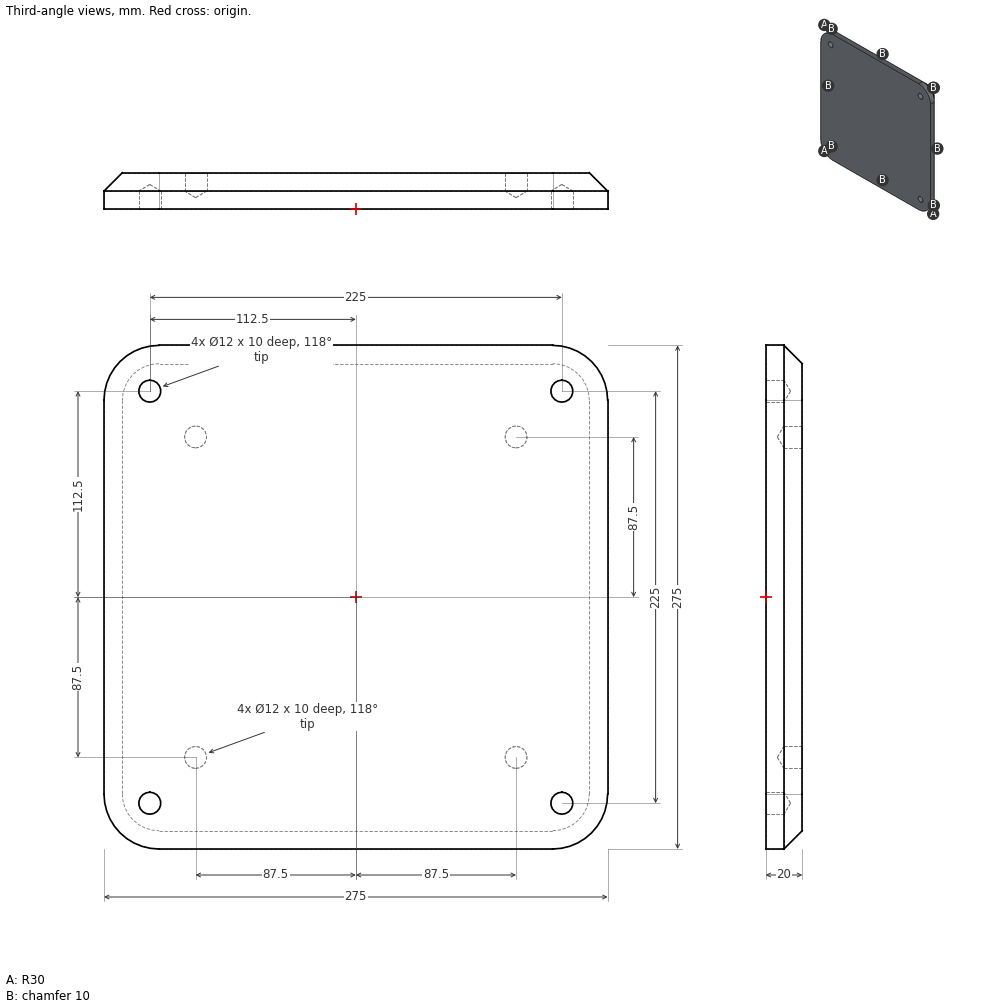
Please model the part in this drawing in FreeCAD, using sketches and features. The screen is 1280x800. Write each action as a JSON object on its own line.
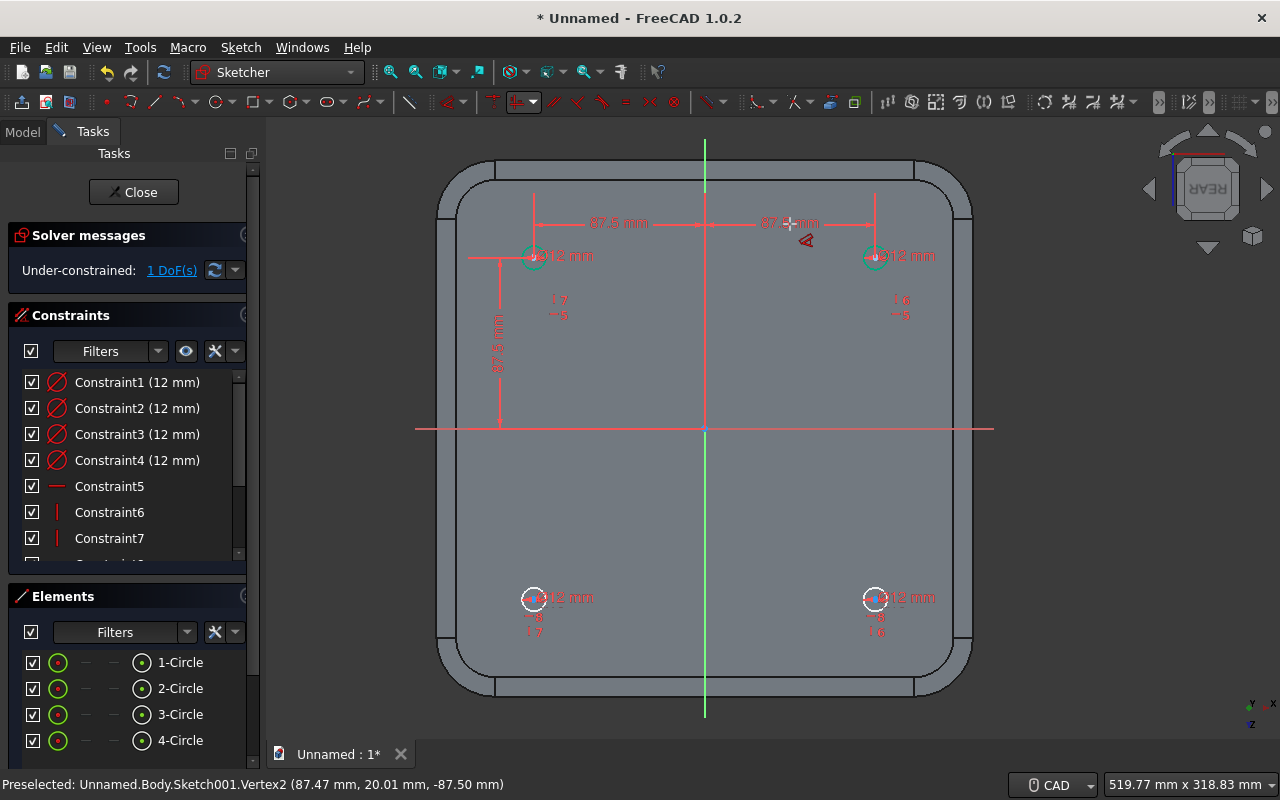
{"action": "left_click", "coordinate": [875, 600]}
{"action": "left_click", "coordinate": [909, 514]}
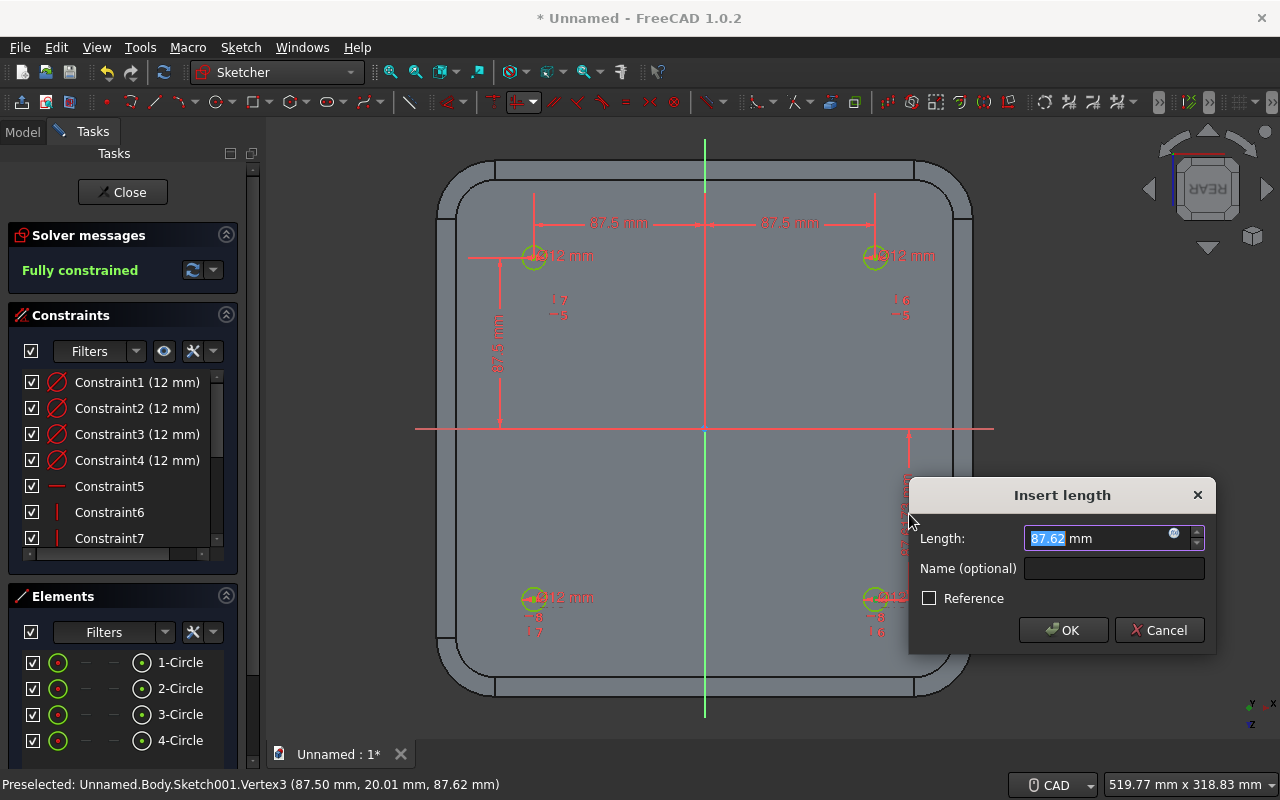
{"action": "type", "text": "87.5"}
{"action": "key", "text": "Return"}
{"action": "key", "text": "Escape"}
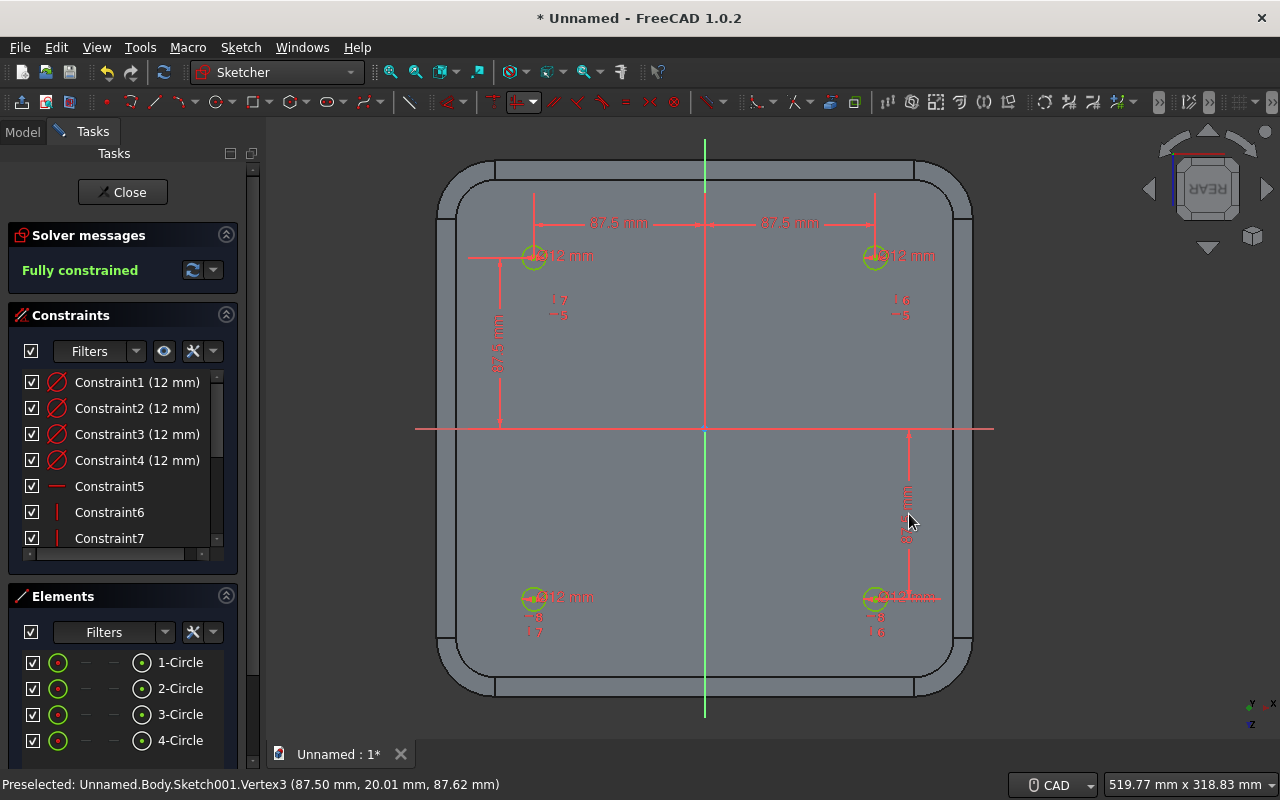
{"action": "left_click", "coordinate": [123, 192]}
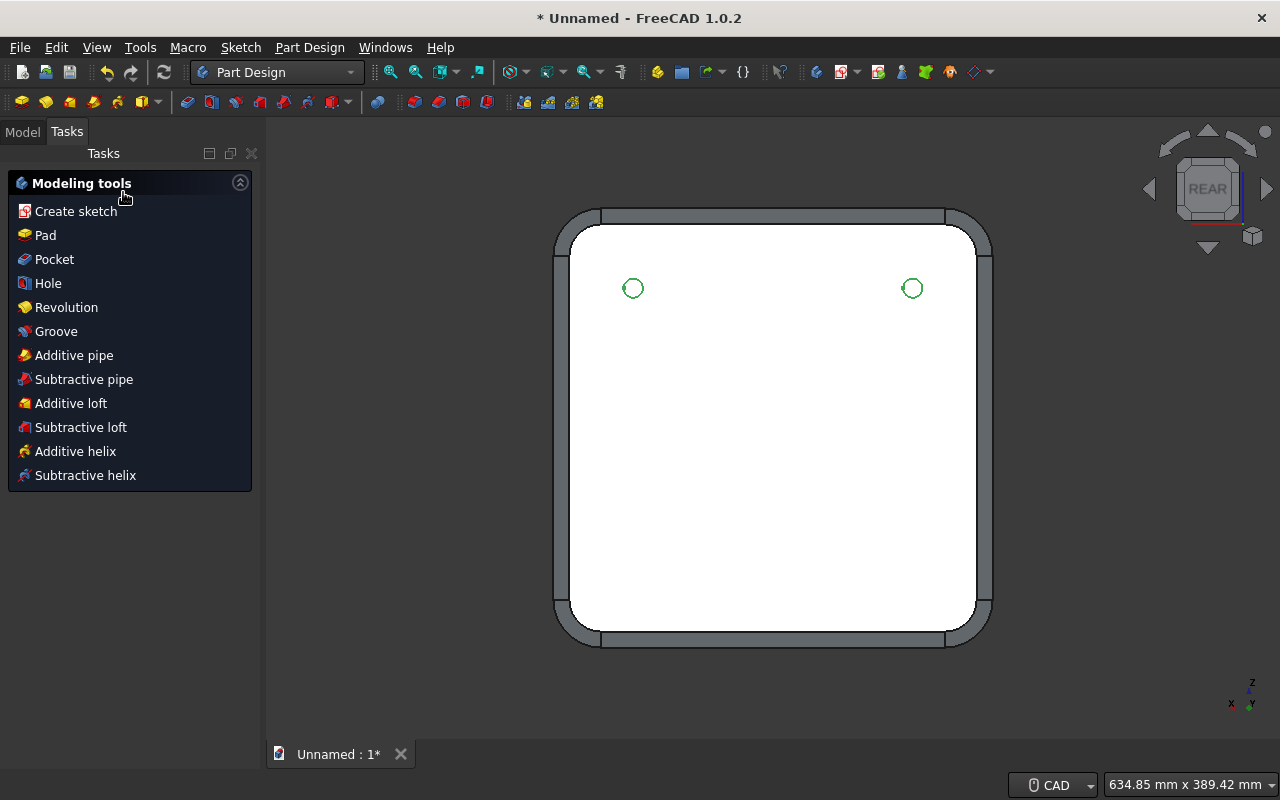
{"action": "left_click", "coordinate": [212, 102]}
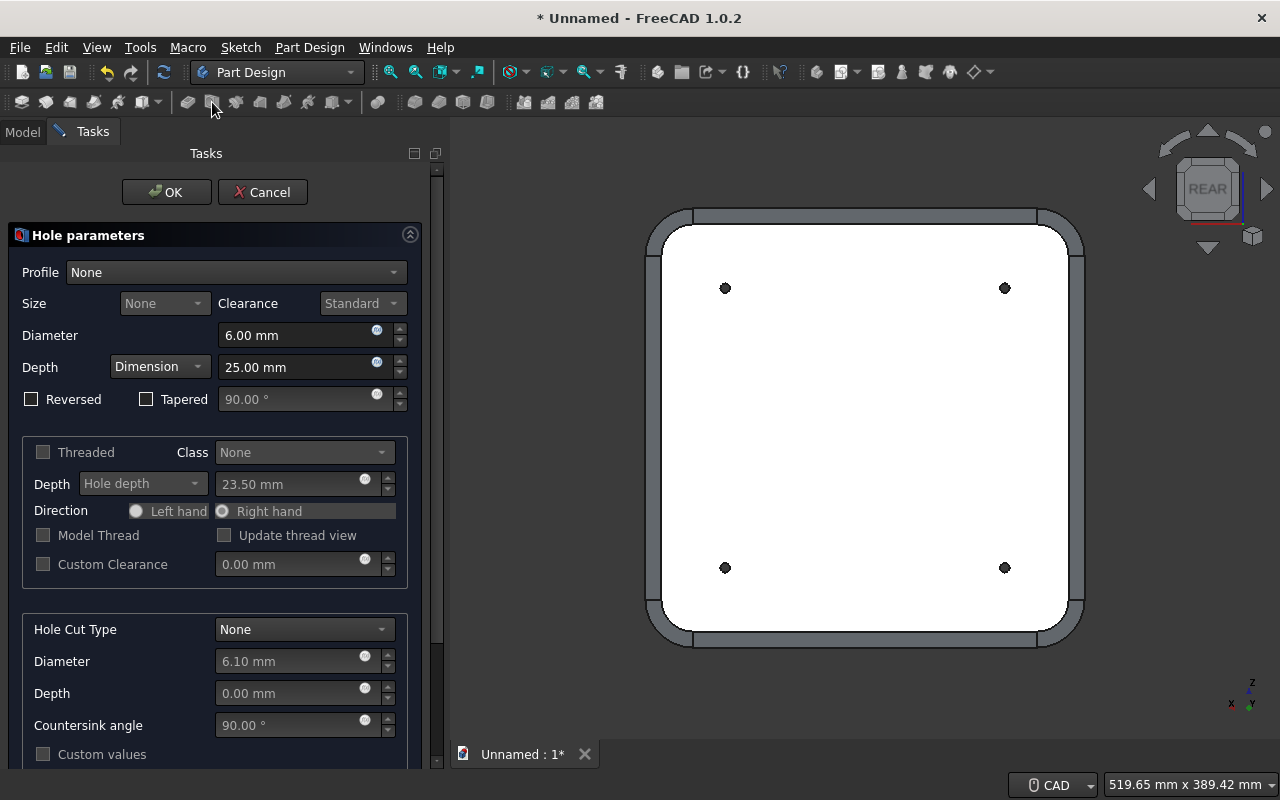
{"action": "triple_click", "coordinate": [305, 335]}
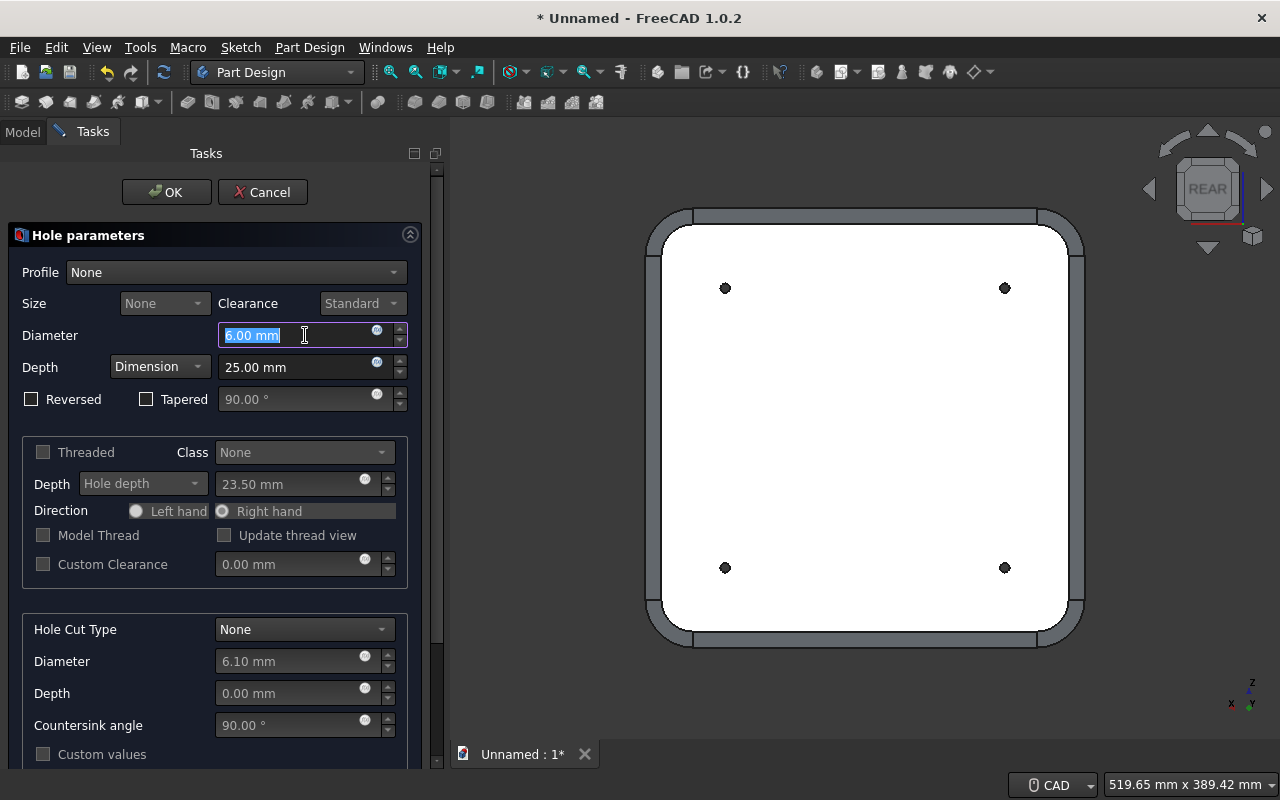
{"action": "type", "text": "12"}
{"action": "key", "text": "Tab"}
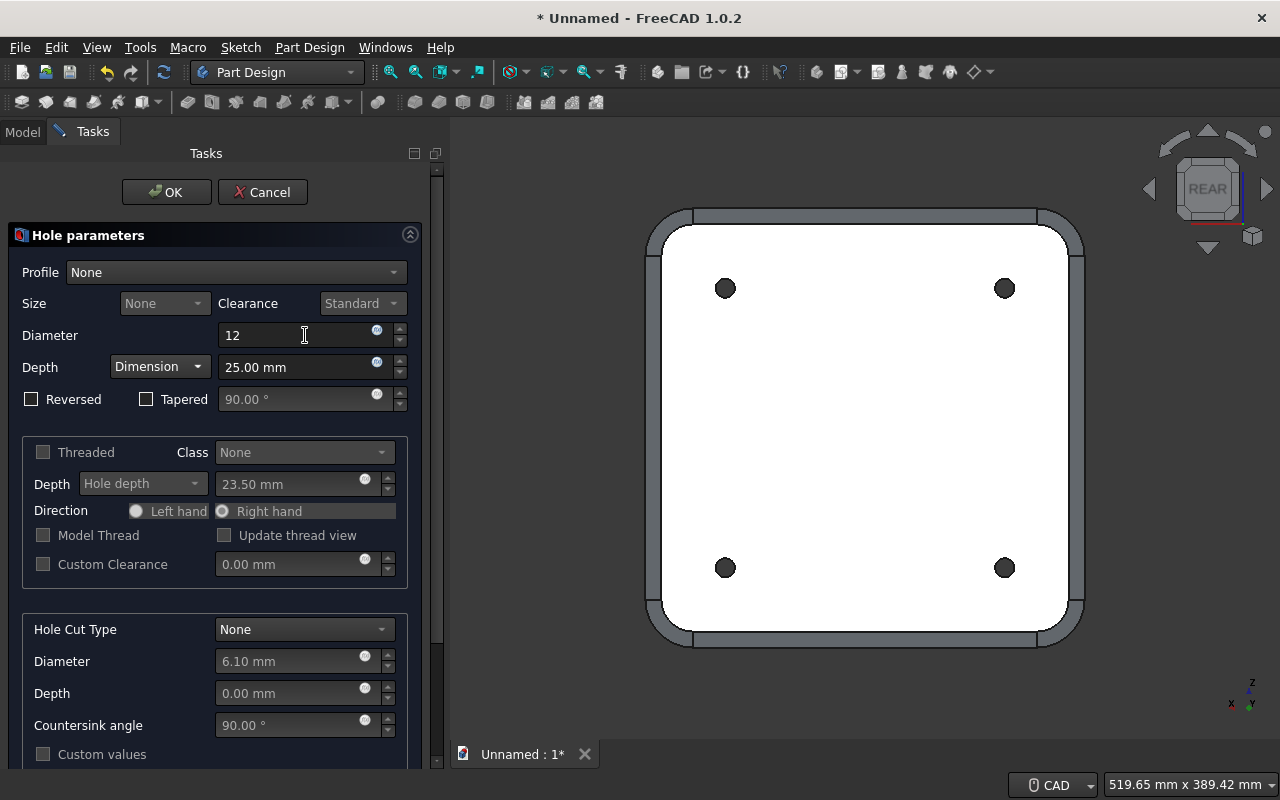
{"action": "triple_click", "coordinate": [305, 367]}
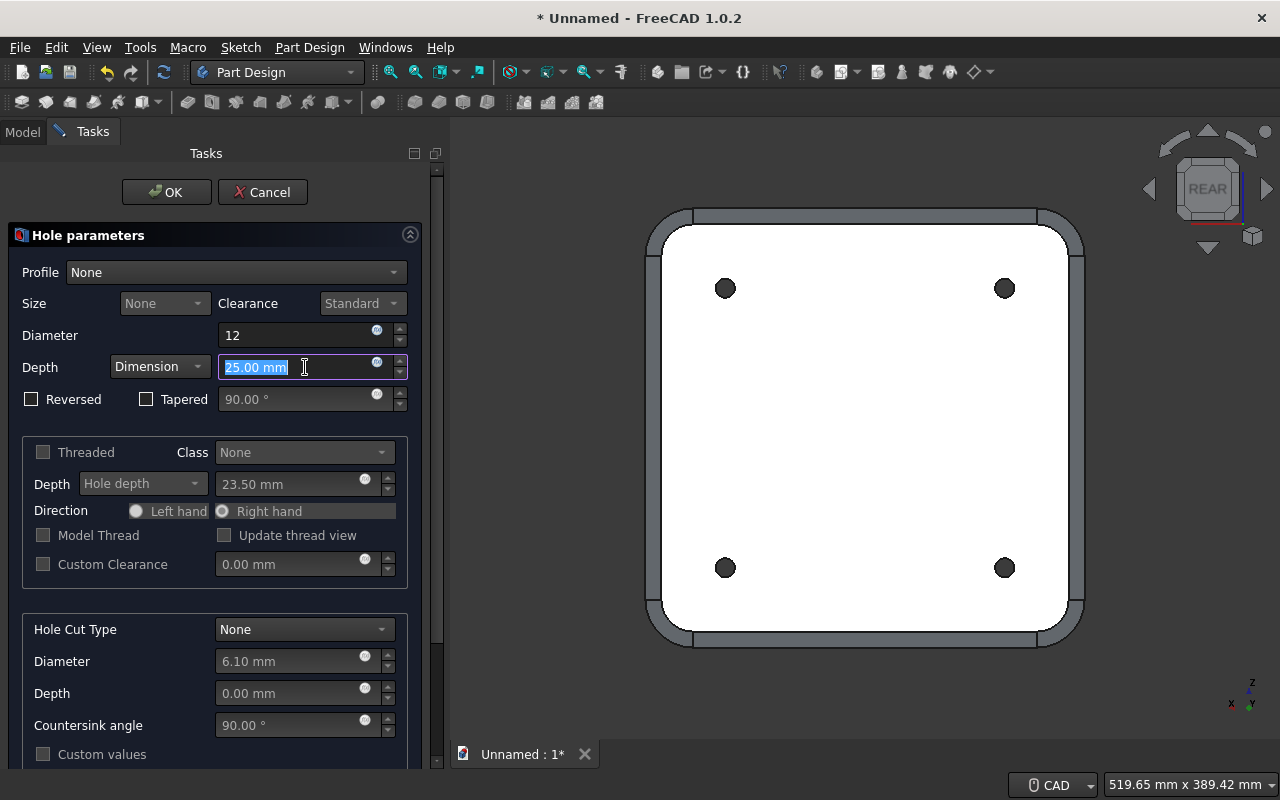
{"action": "type", "text": "10"}
{"action": "key", "text": "Tab"}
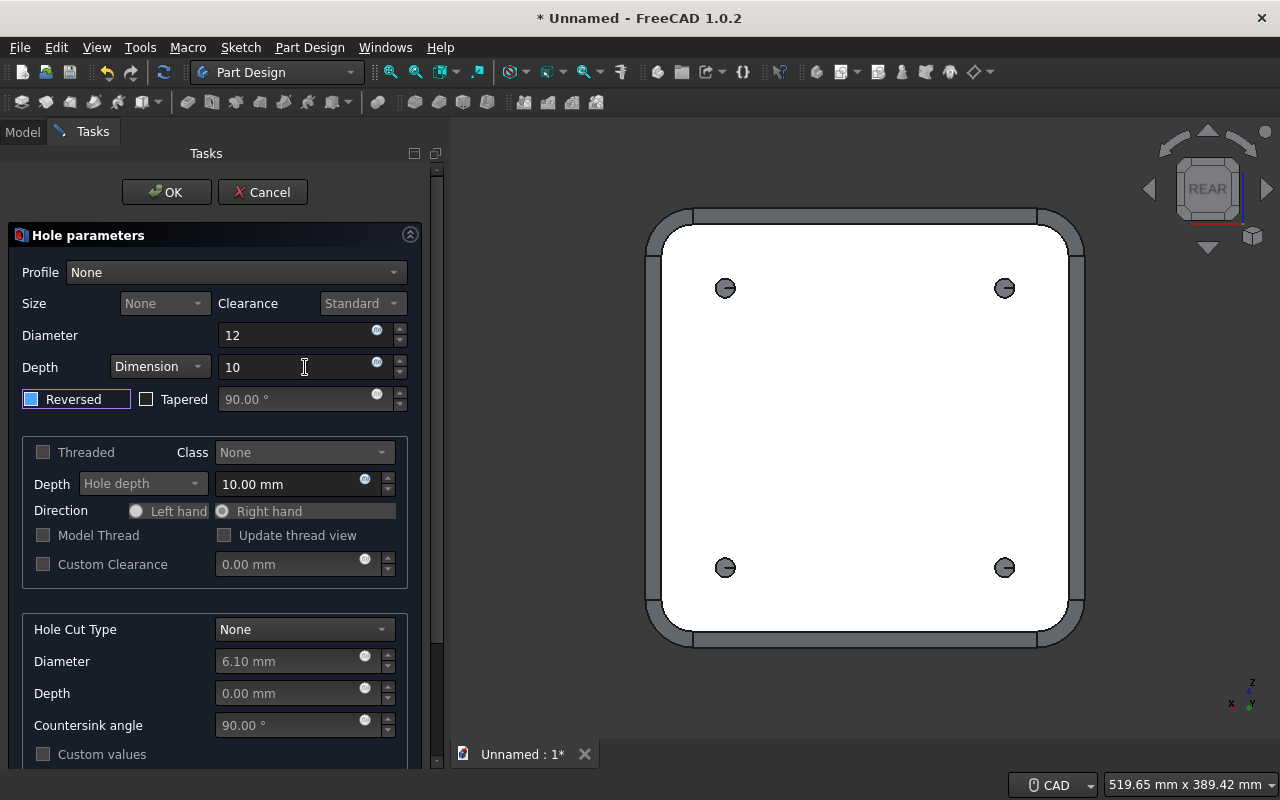
{"action": "left_click", "coordinate": [167, 192]}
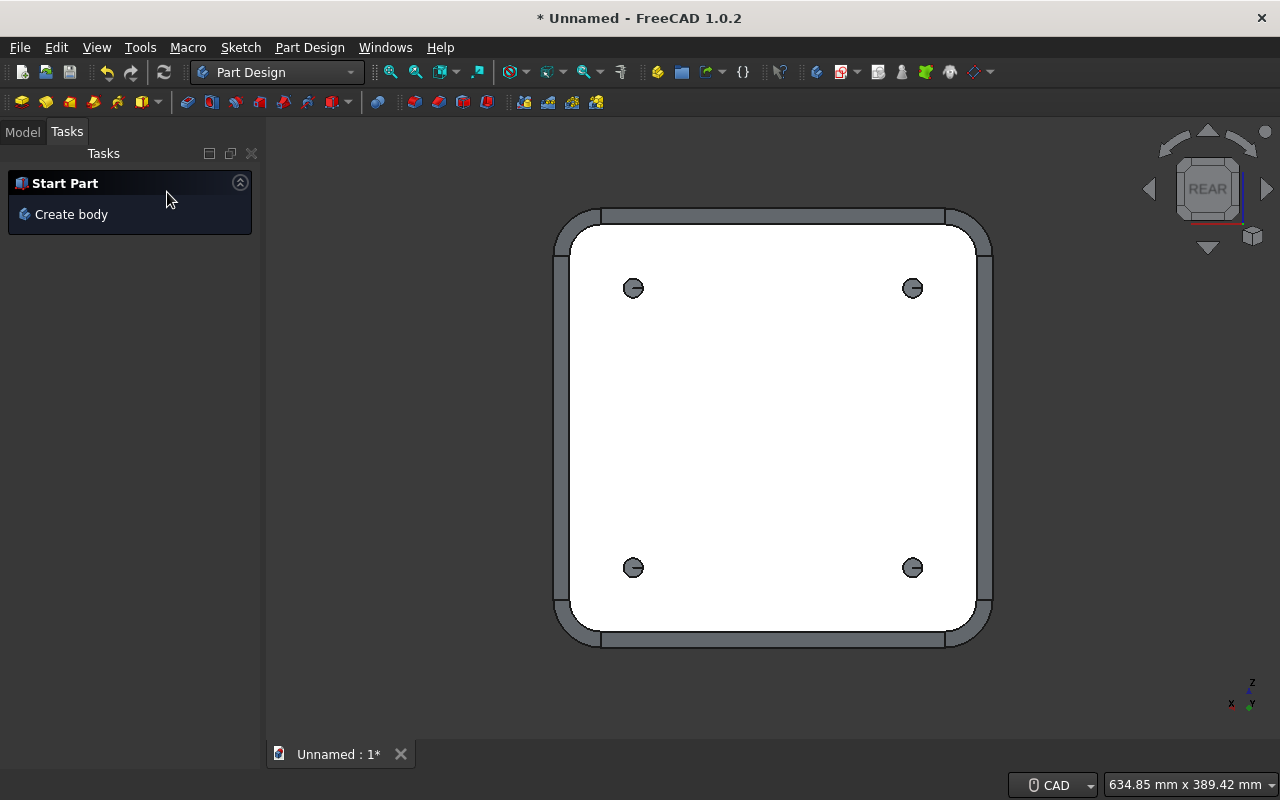
{"action": "key", "text": "0"}